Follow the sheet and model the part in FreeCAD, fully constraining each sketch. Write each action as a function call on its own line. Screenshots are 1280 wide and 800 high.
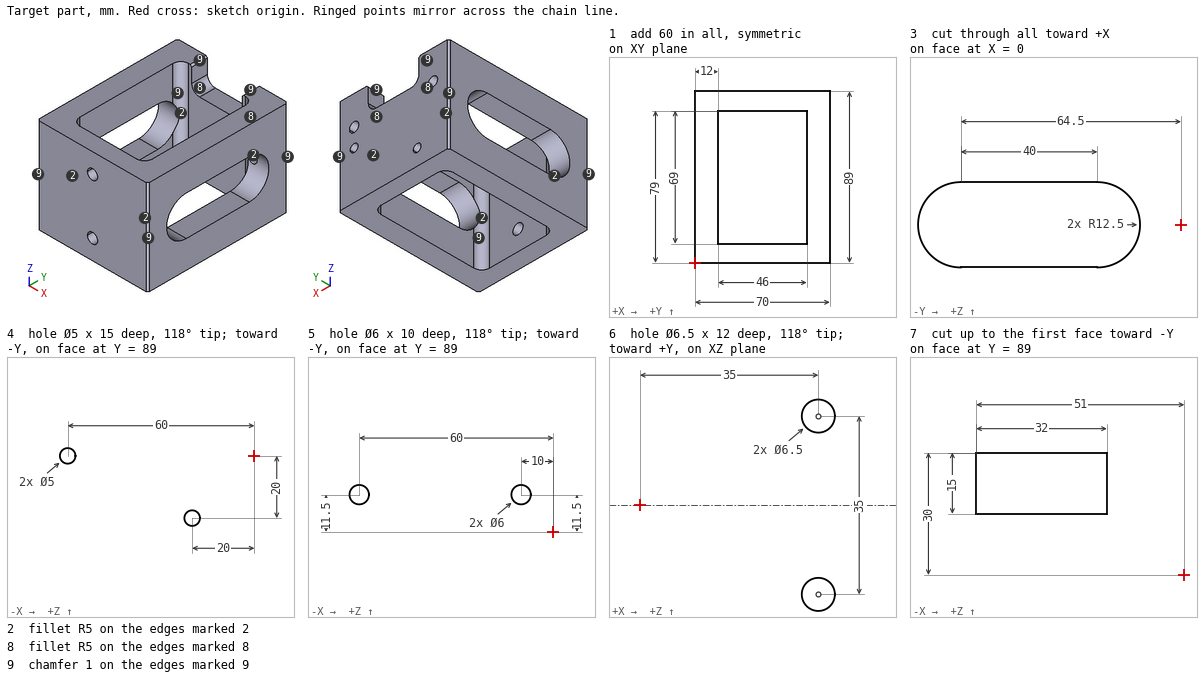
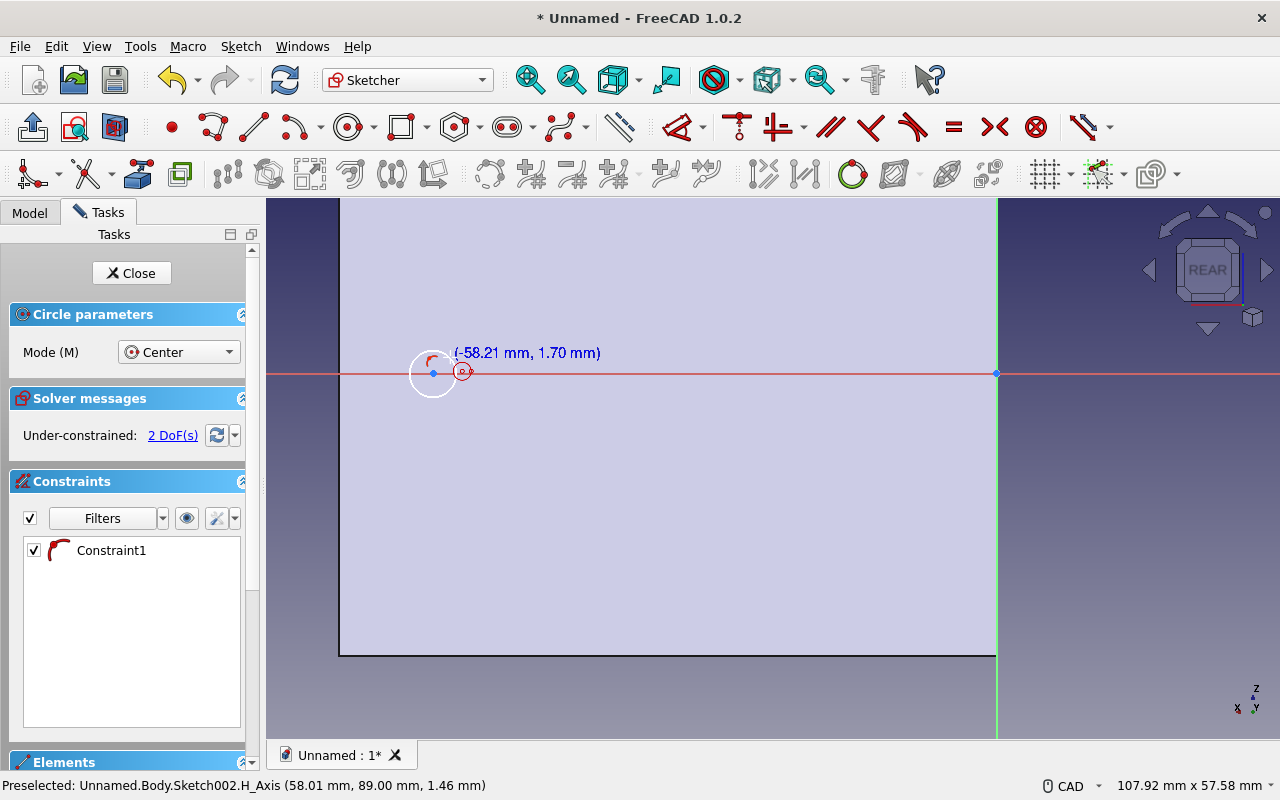
click(809, 562)
click(826, 545)
key(Escape)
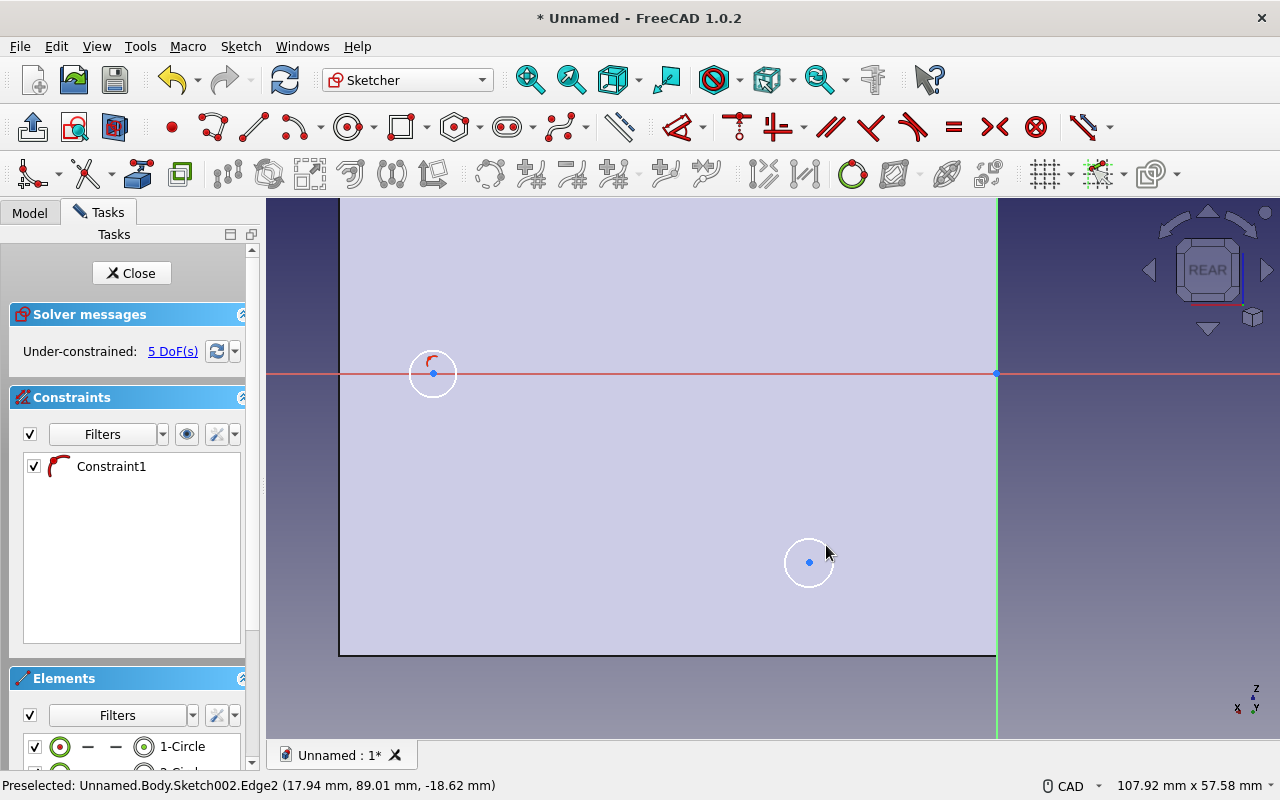
click(449, 357)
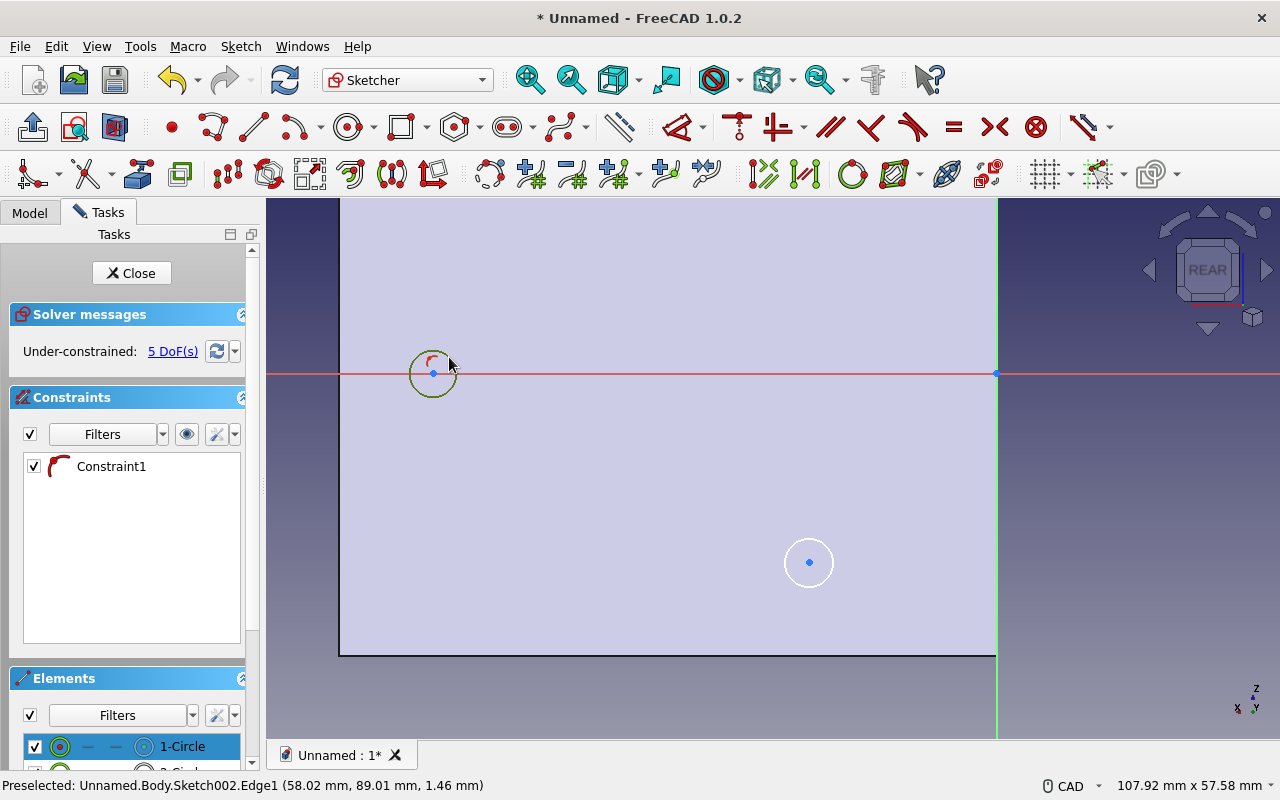
click(826, 546)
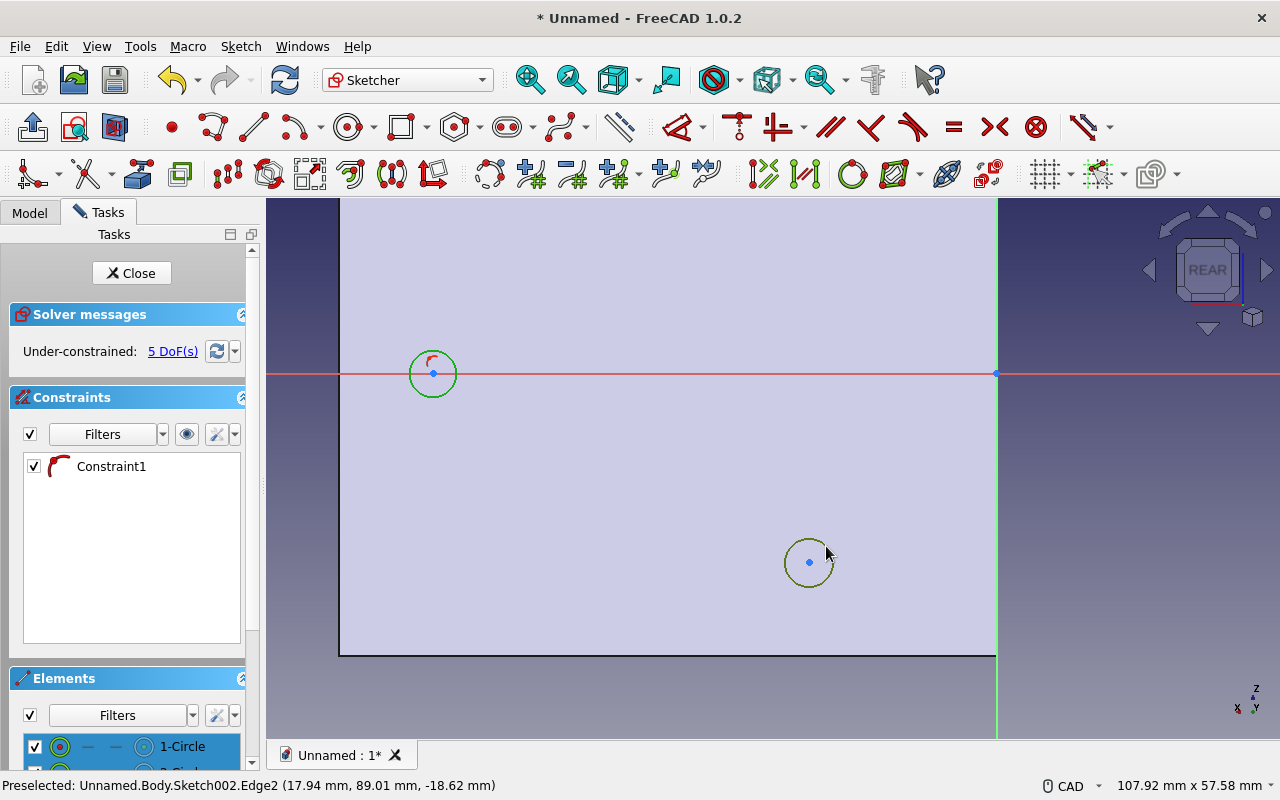
click(954, 128)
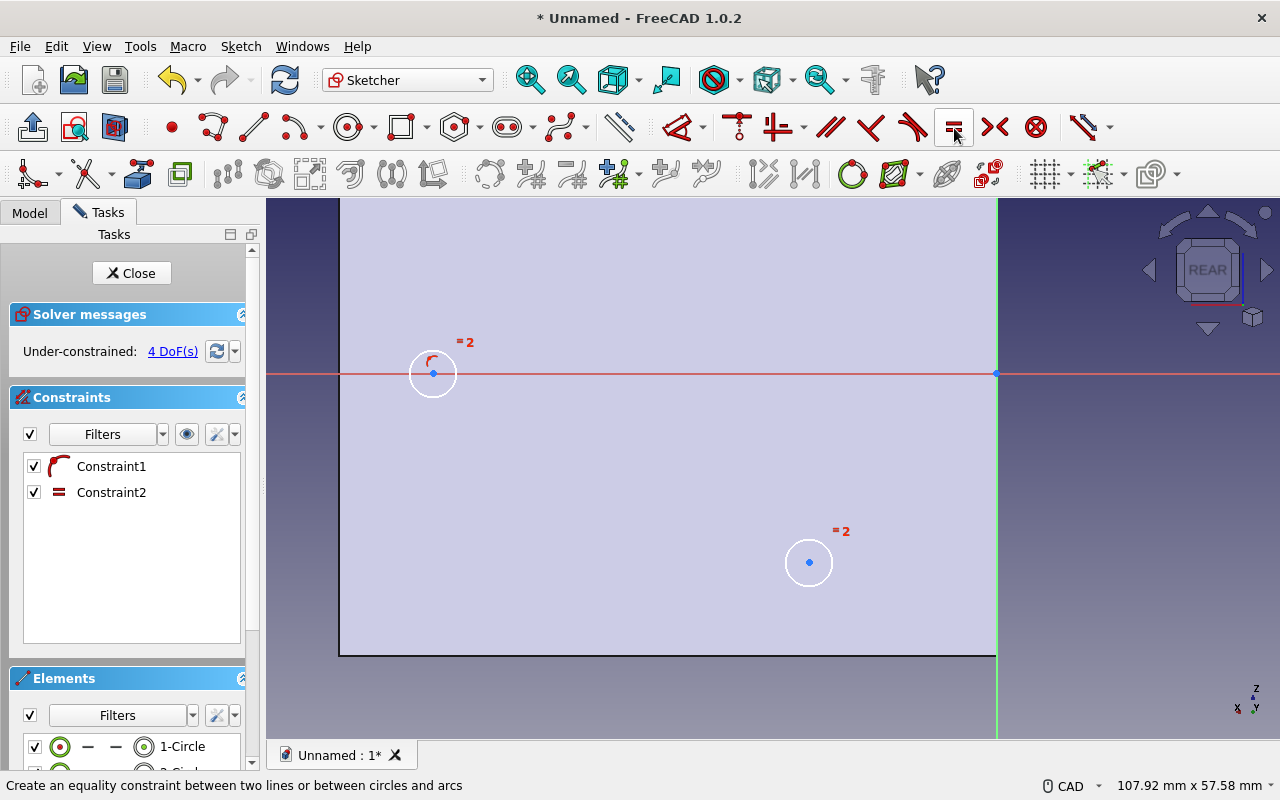
click(676, 128)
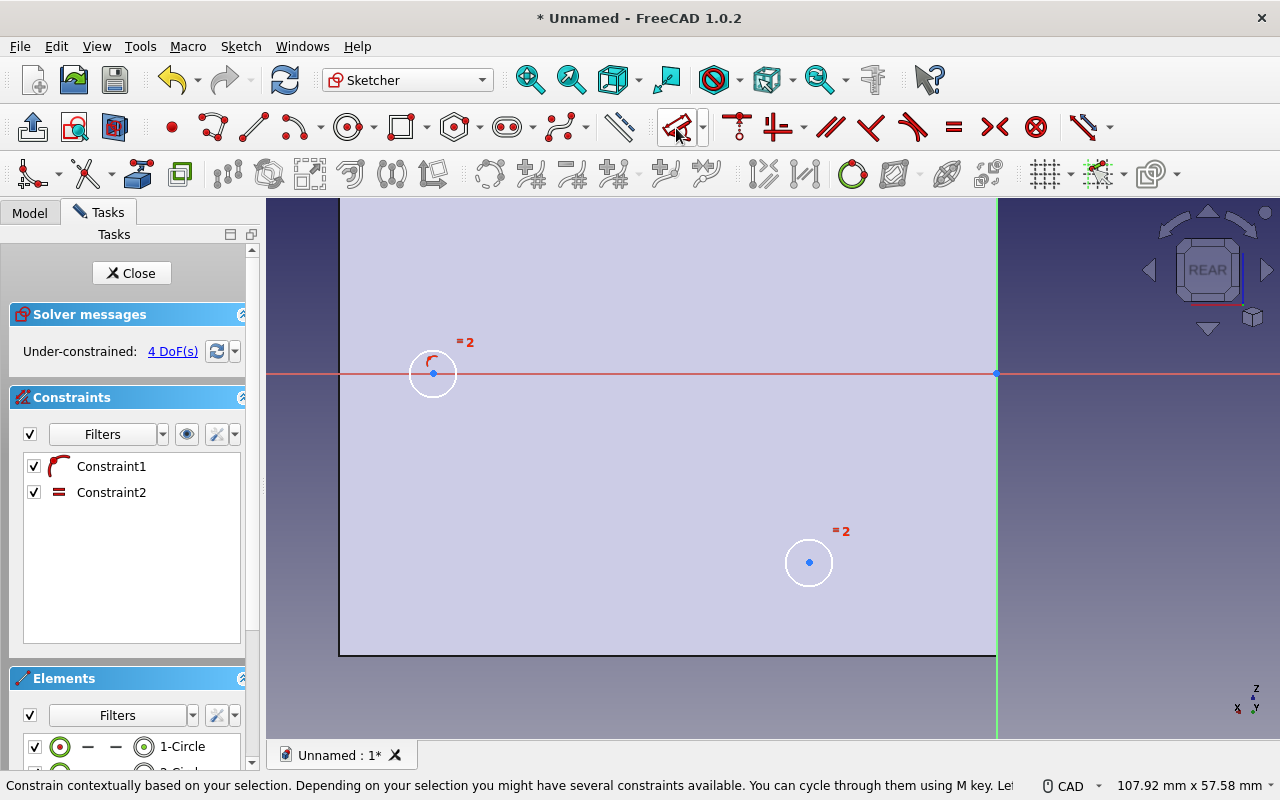
click(449, 357)
click(471, 334)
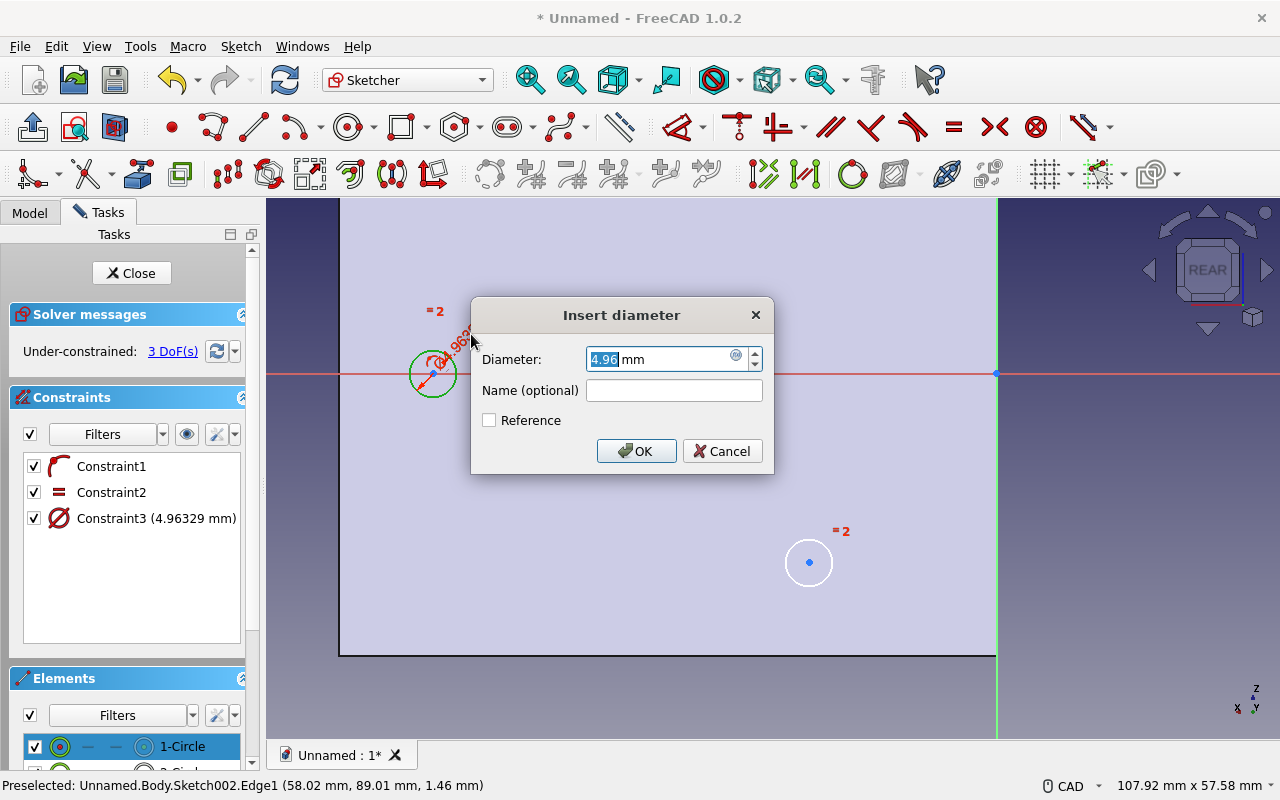
text(5)
key(Return)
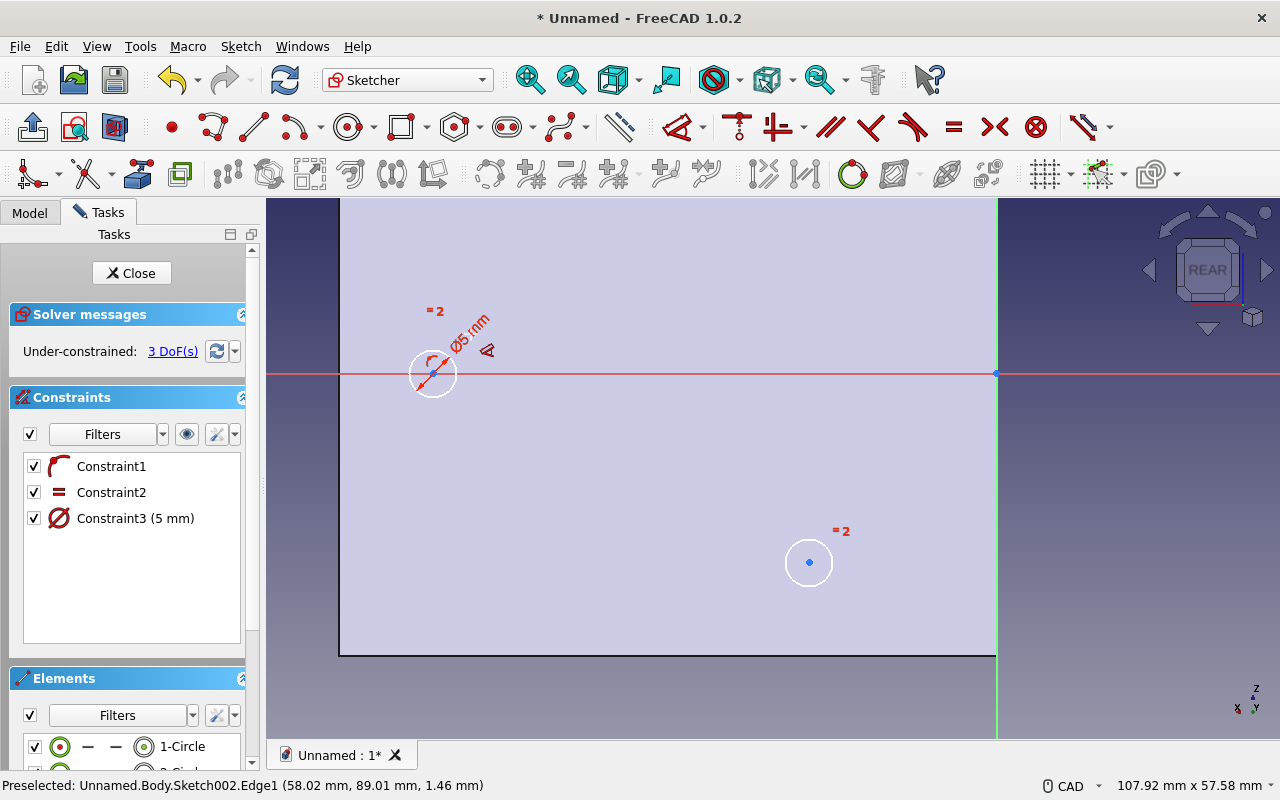
click(433, 374)
click(715, 340)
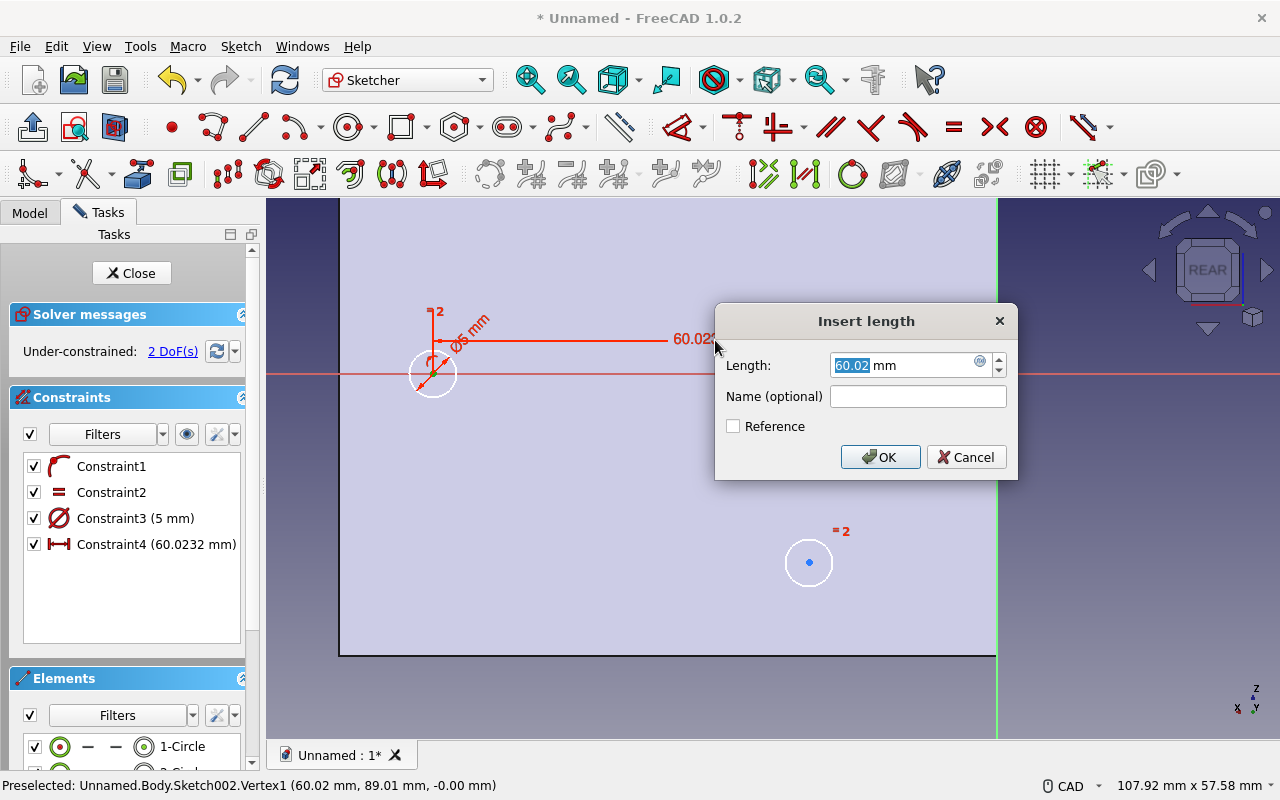
text(60)
key(Return)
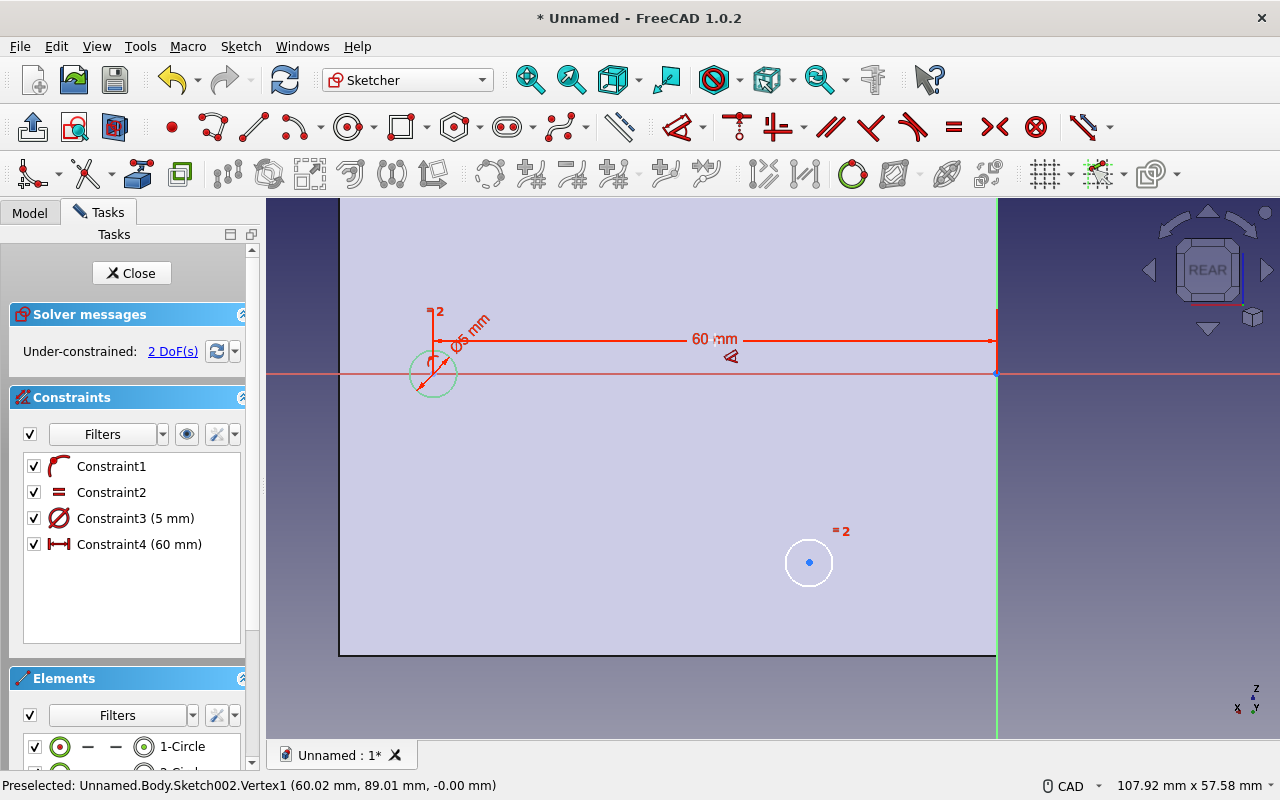
click(809, 563)
click(903, 597)